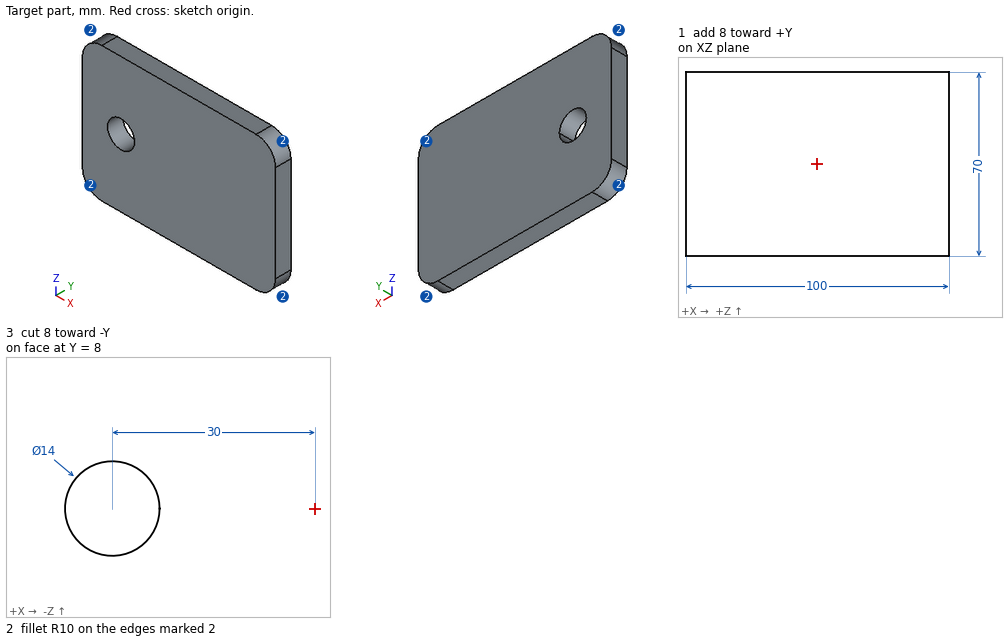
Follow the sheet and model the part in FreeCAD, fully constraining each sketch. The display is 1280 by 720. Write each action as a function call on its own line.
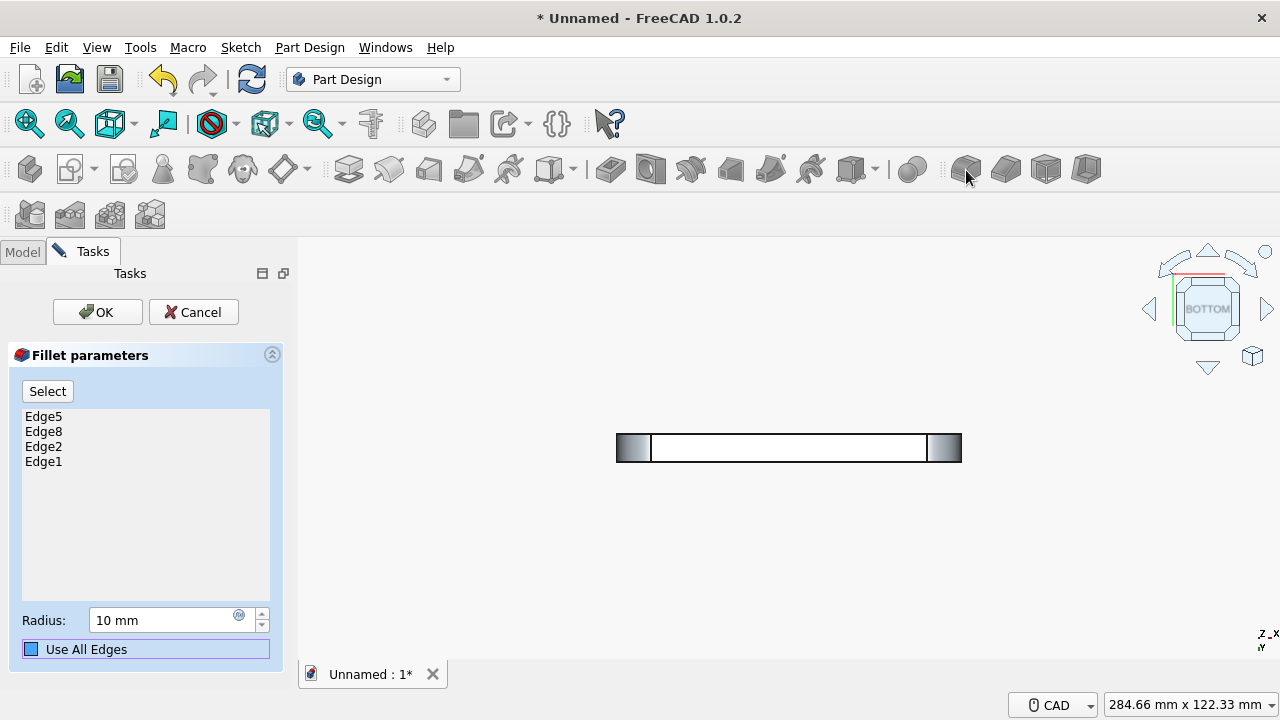
click(98, 312)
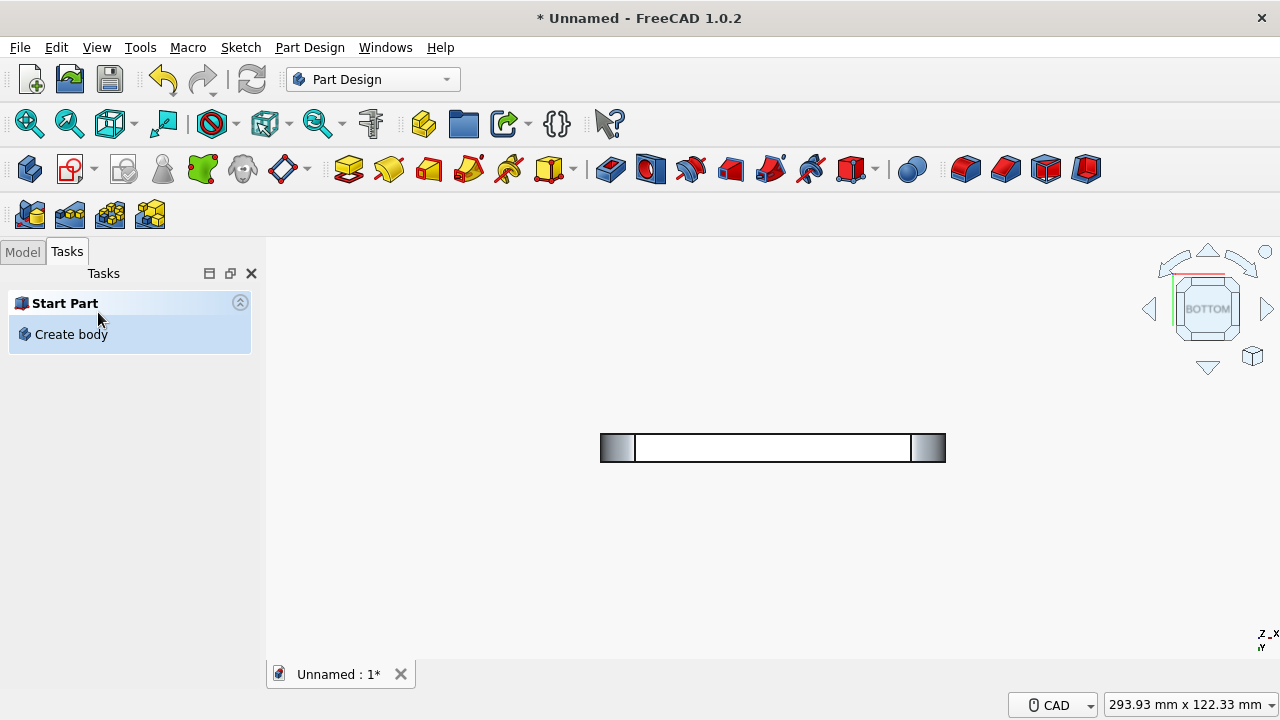
click(30, 124)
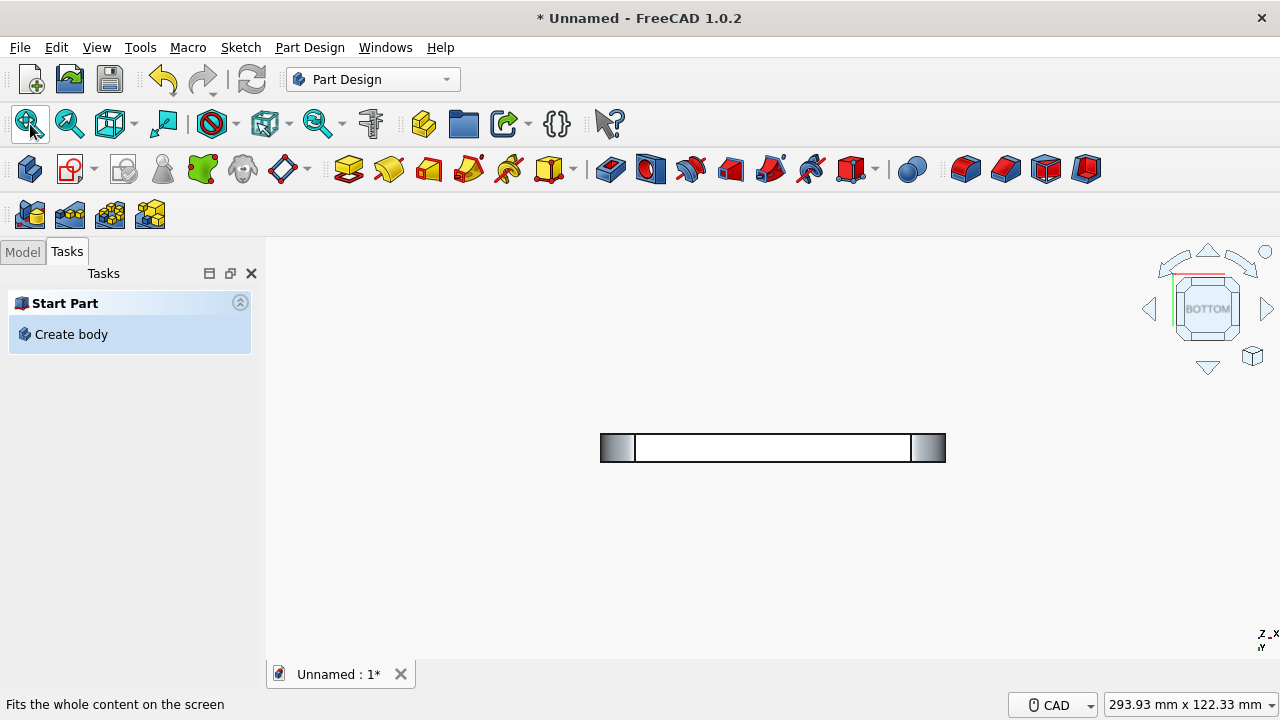
key(4)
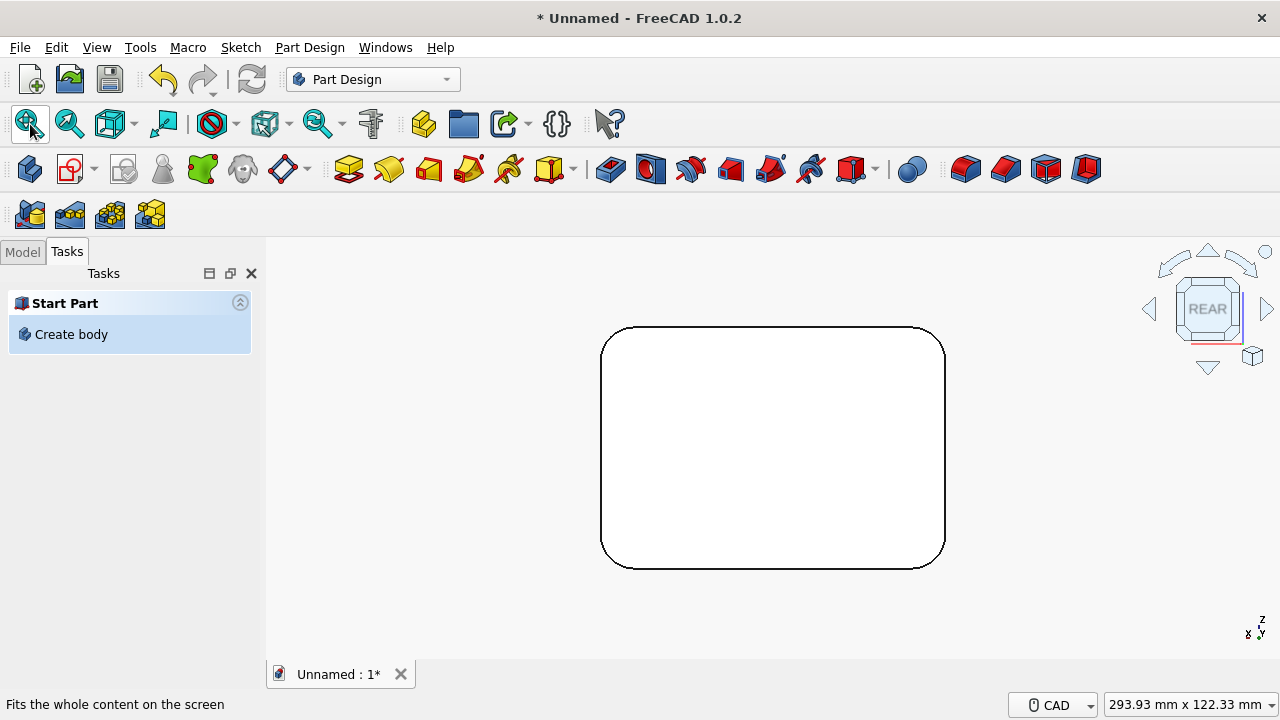
click(724, 447)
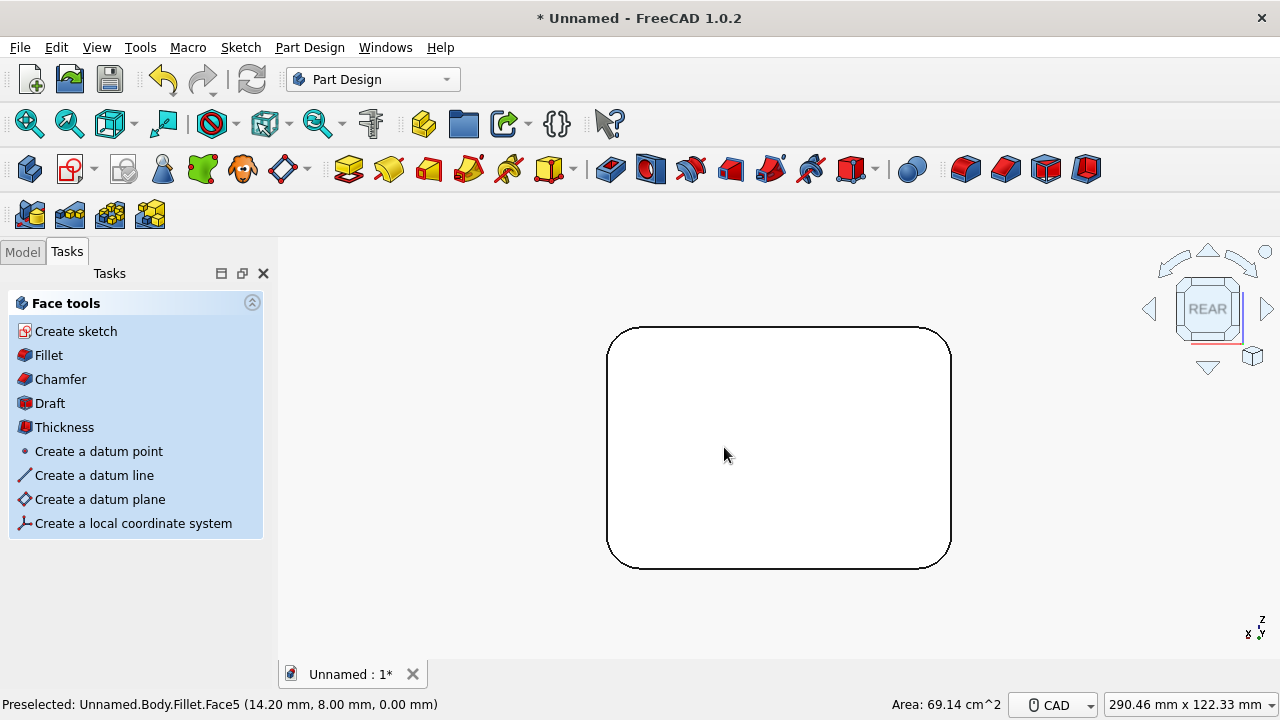
click(70, 170)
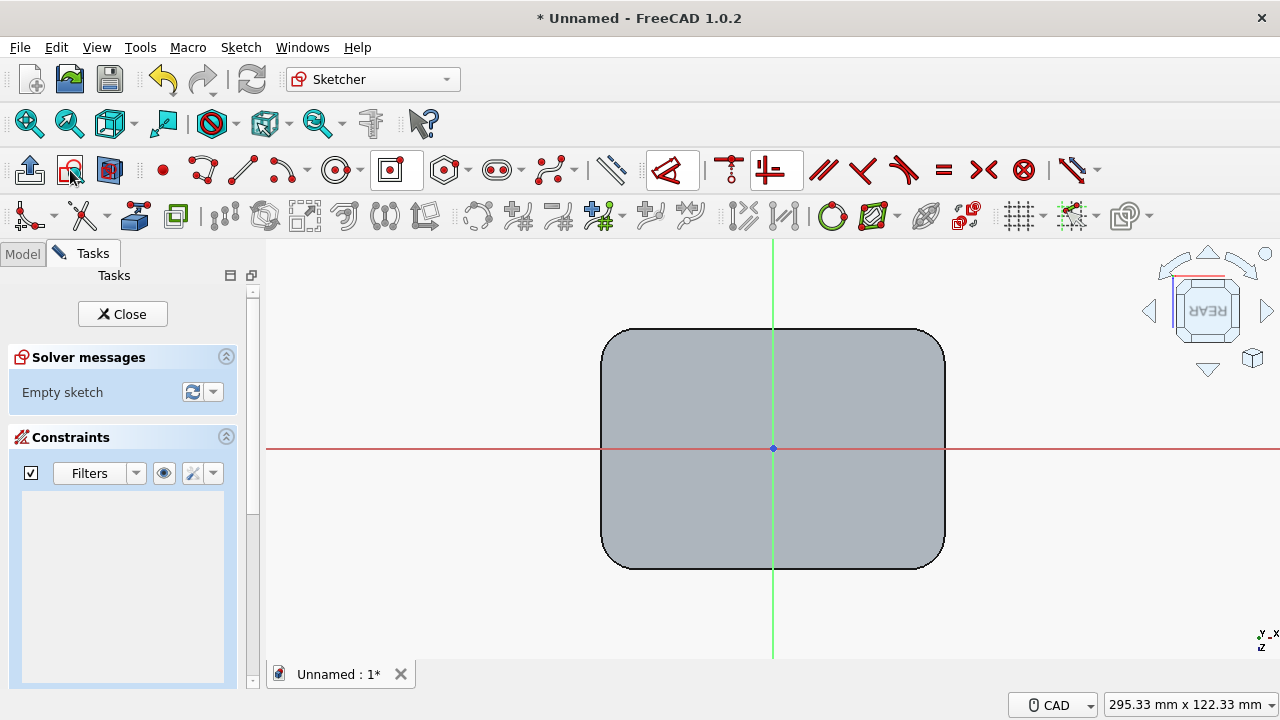
scroll(661, 449, up, 8)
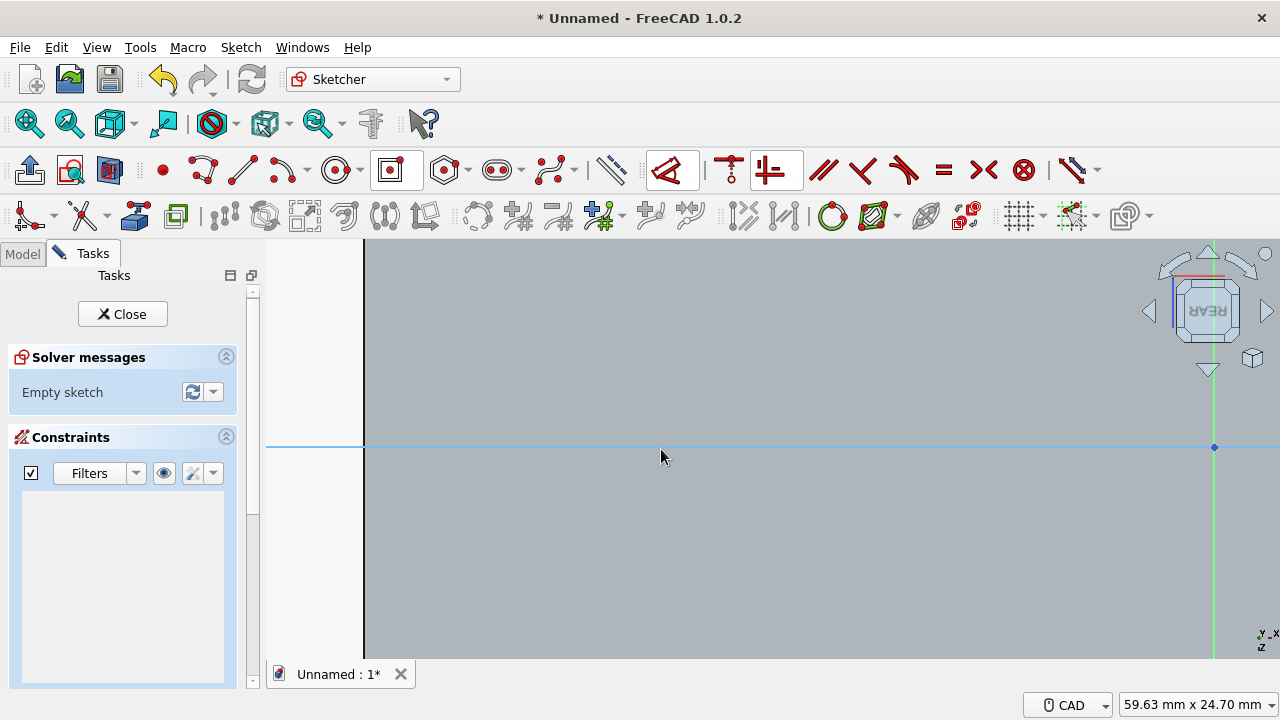
click(336, 170)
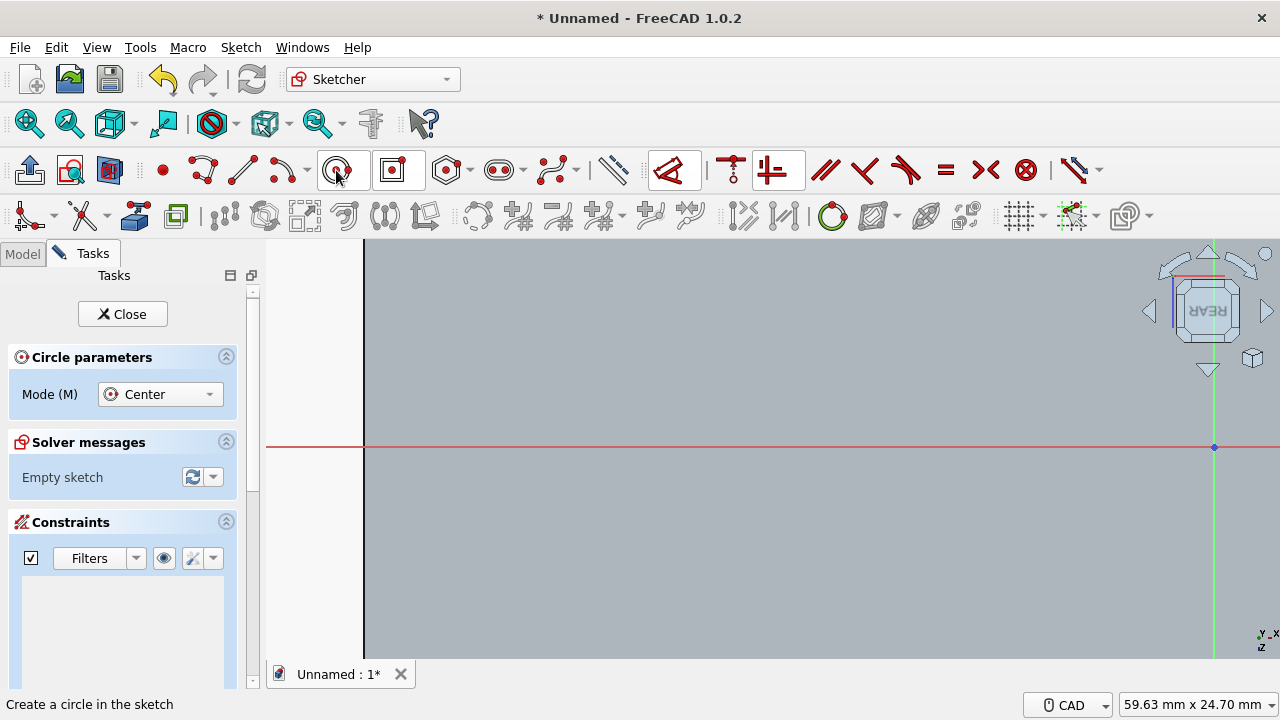
click(704, 447)
click(788, 363)
key(Escape)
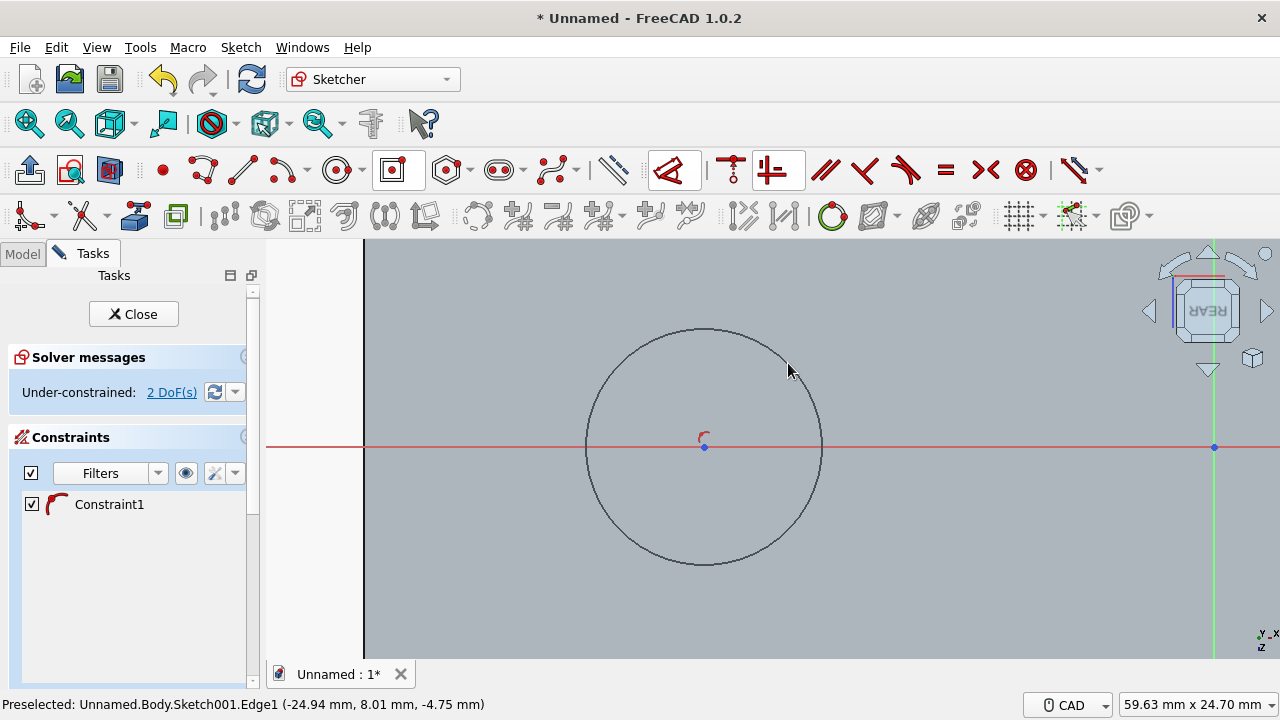
click(787, 363)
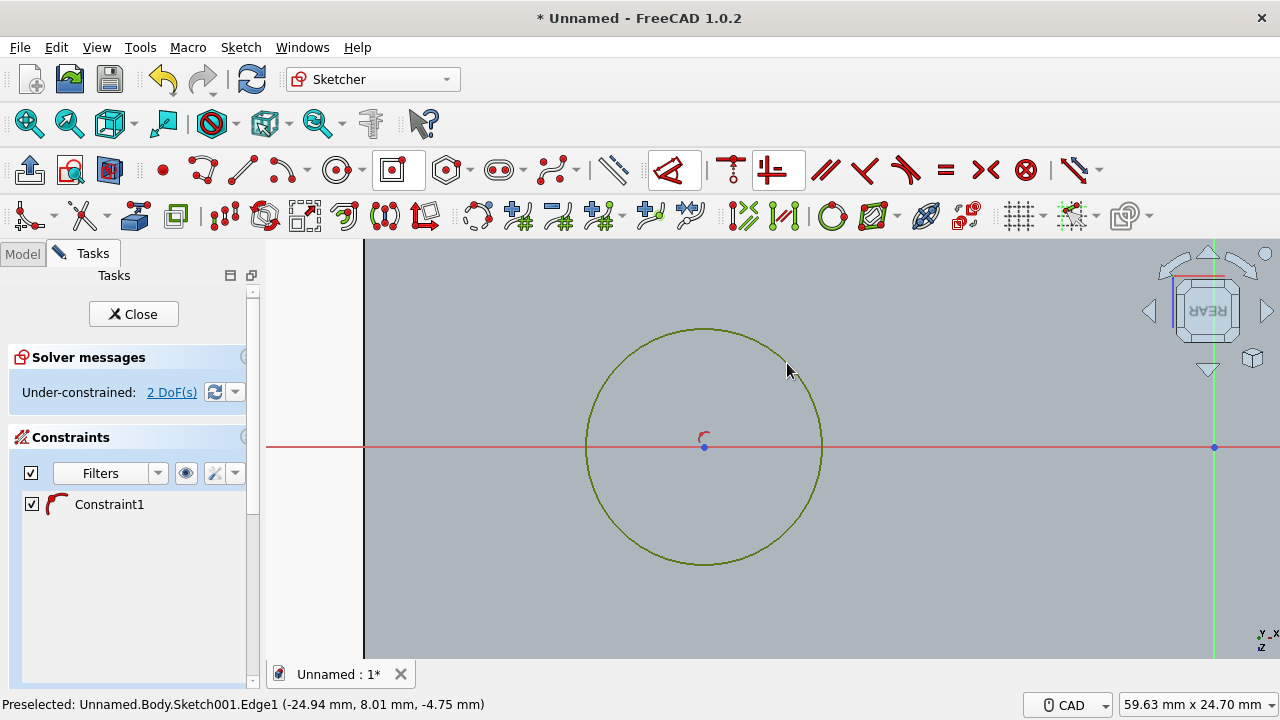
key(k)
key(o)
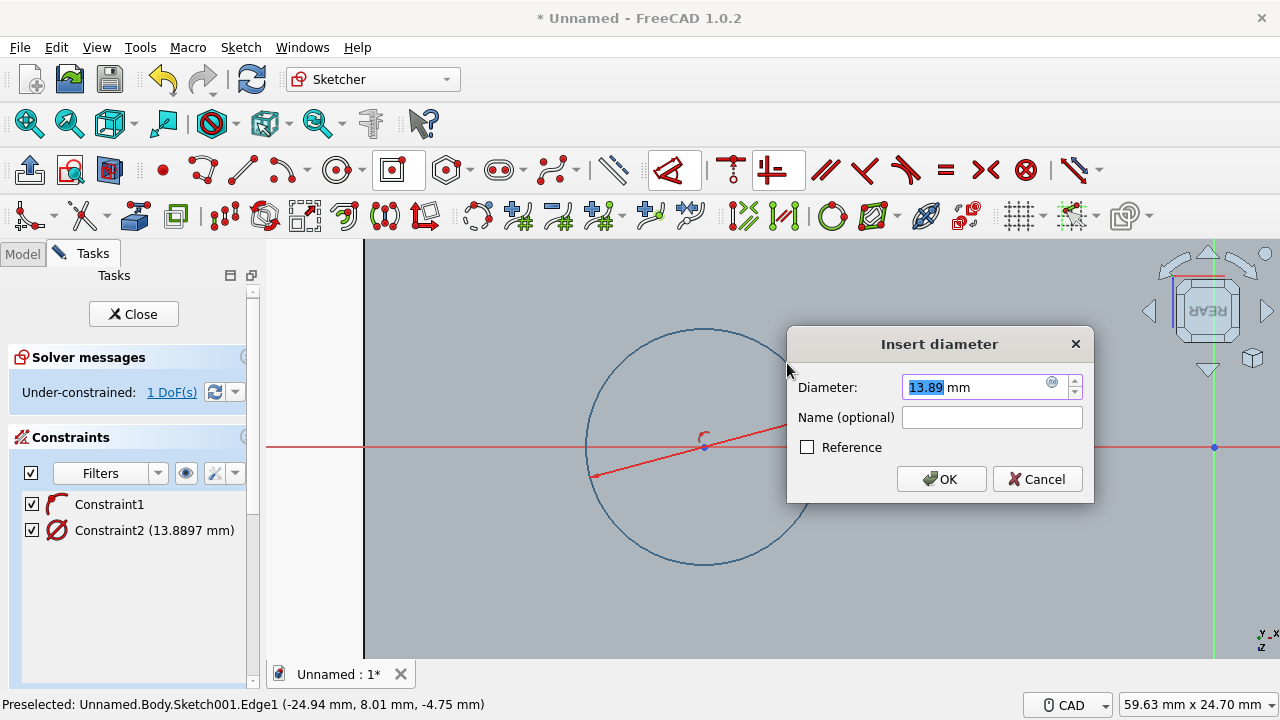
text(14)
key(Return)